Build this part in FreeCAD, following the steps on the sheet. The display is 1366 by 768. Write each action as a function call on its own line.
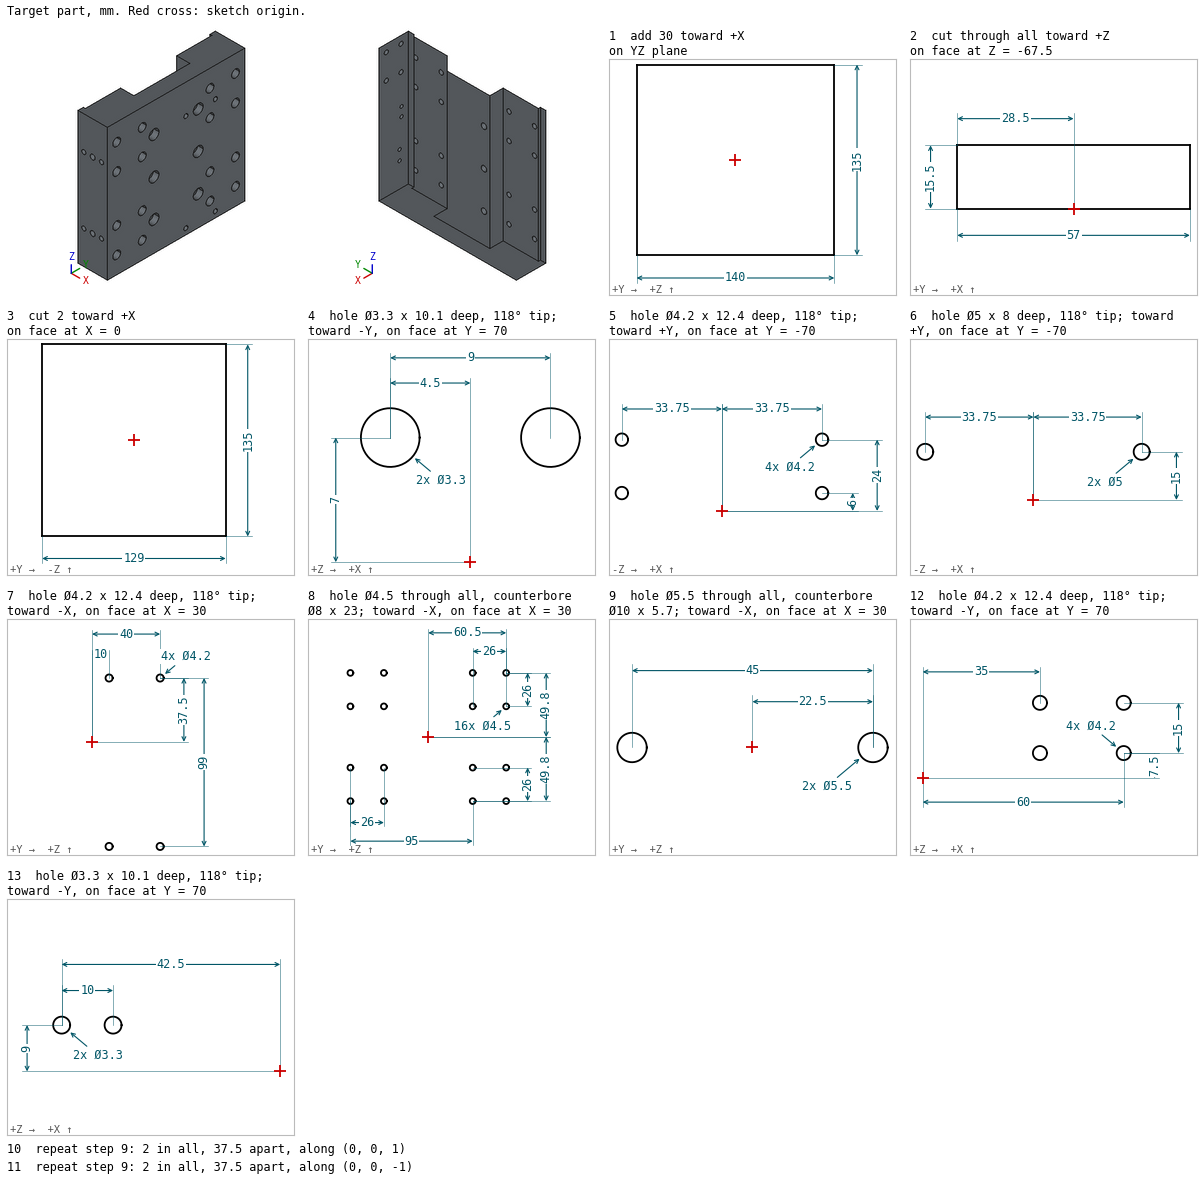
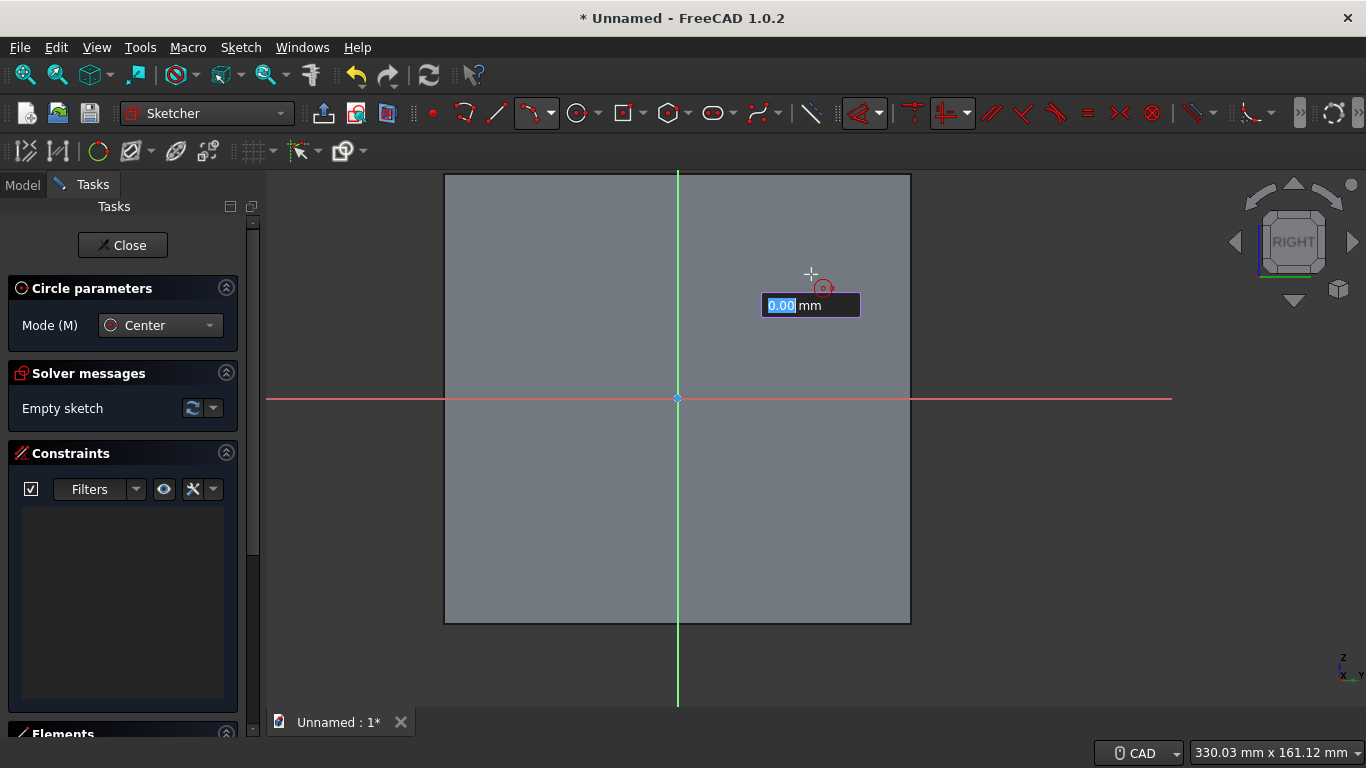
scroll(816, 269, up, 5)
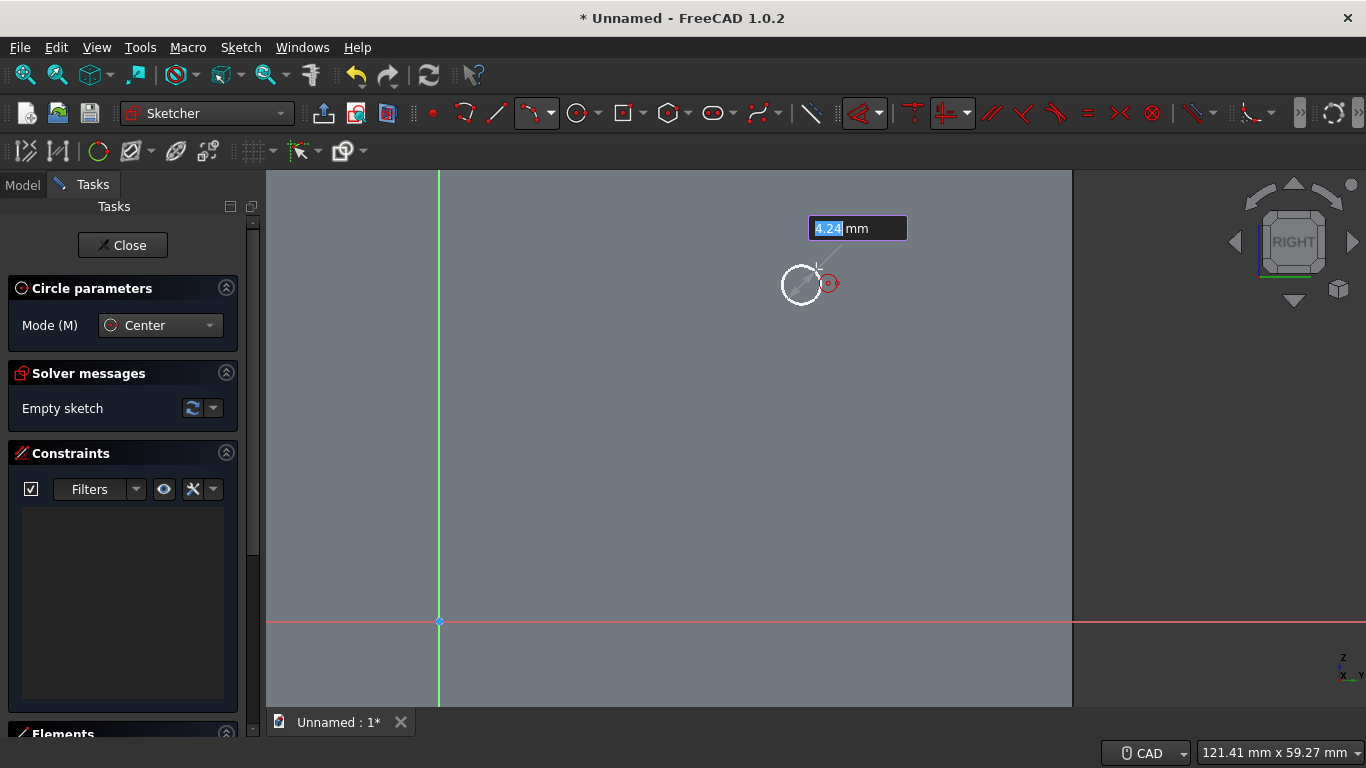
click(815, 268)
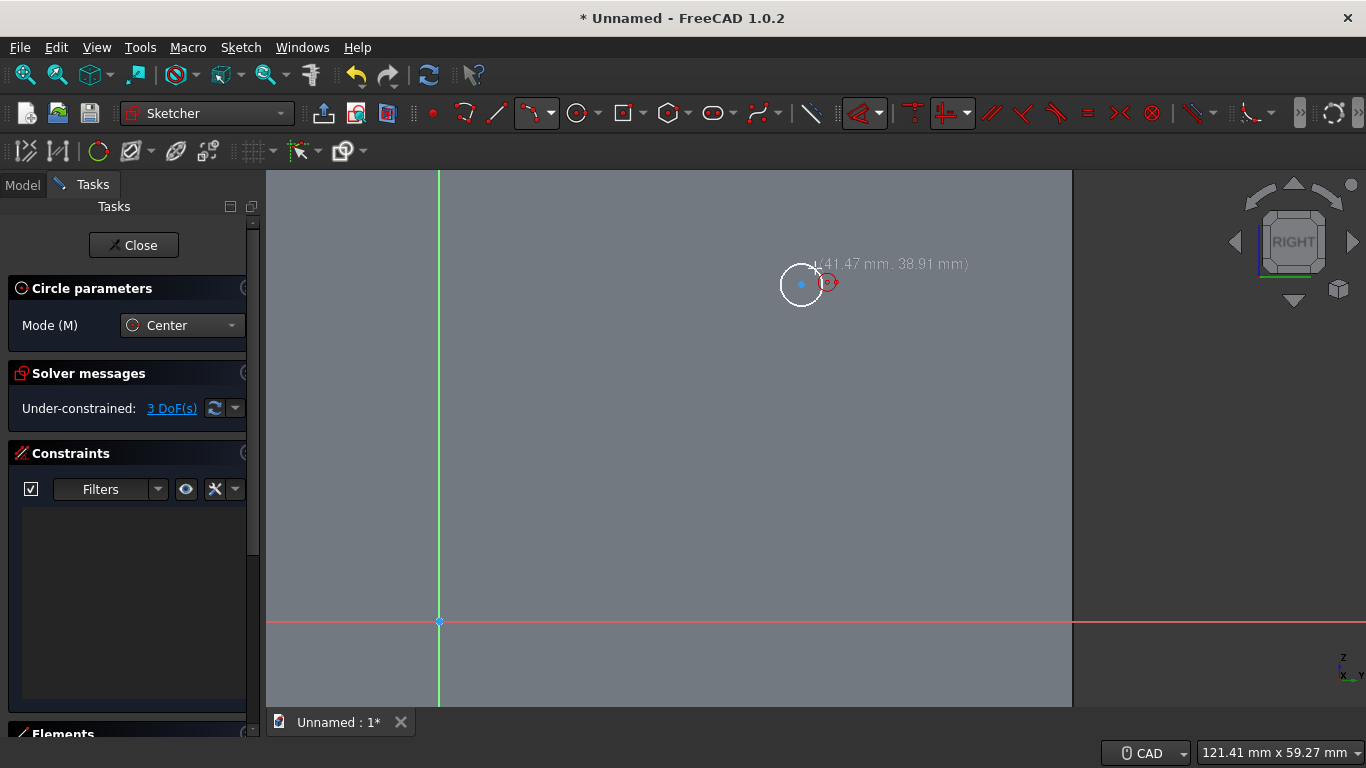
click(530, 282)
click(543, 268)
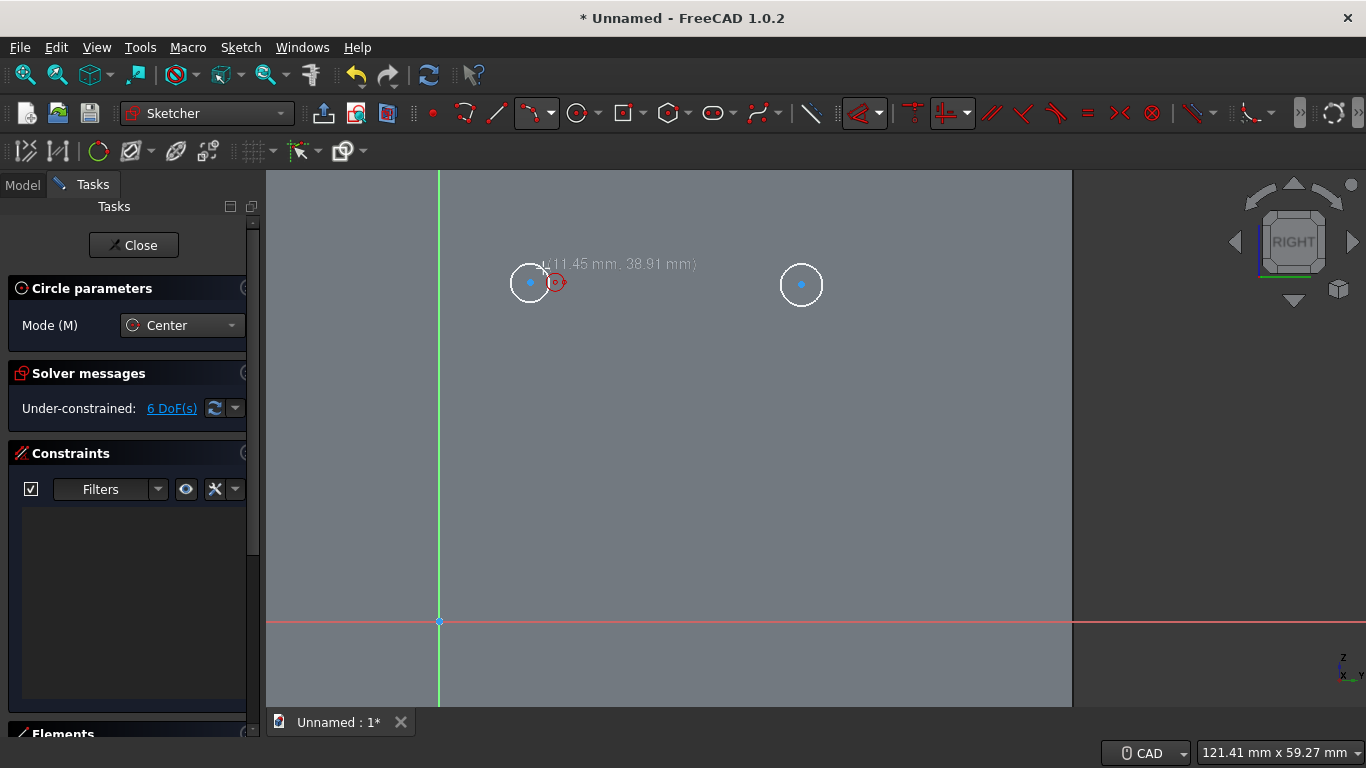
scroll(816, 269, down, 5)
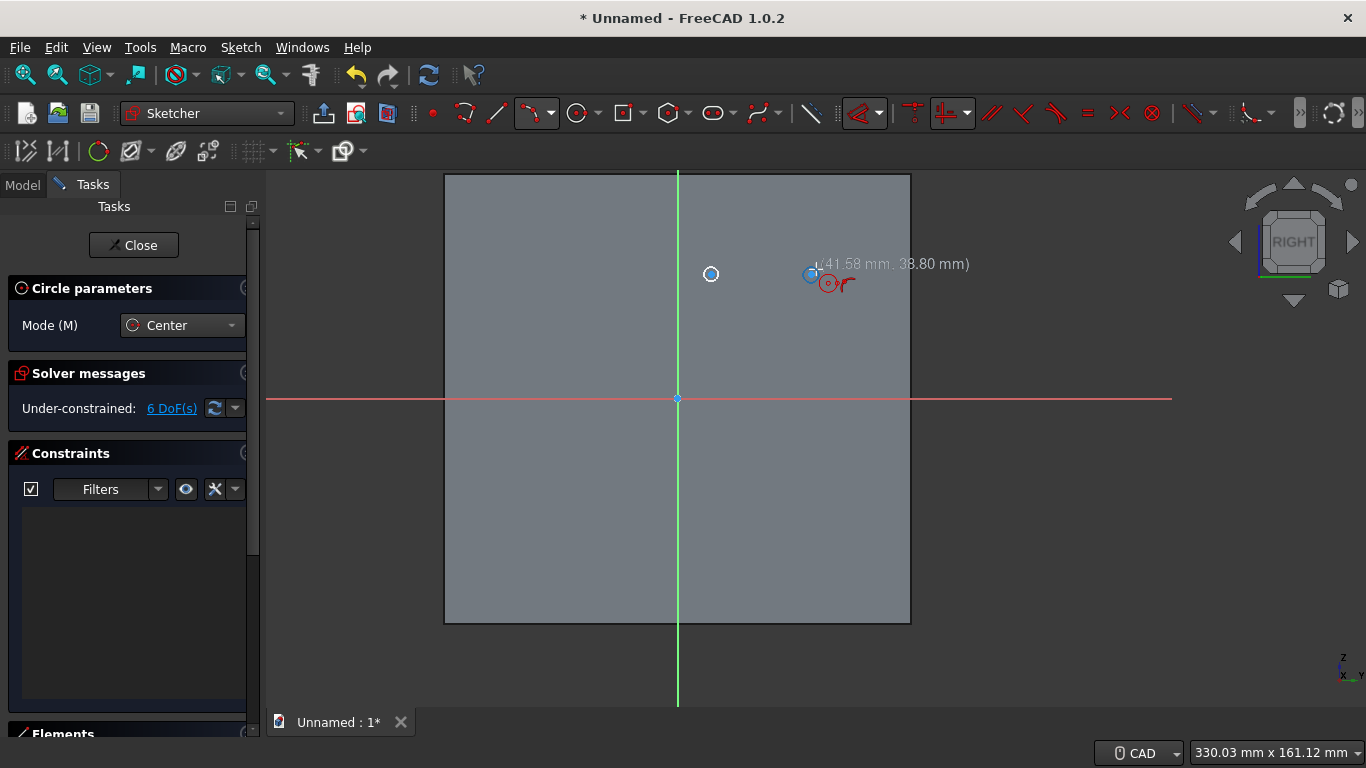
scroll(811, 604, up, 6)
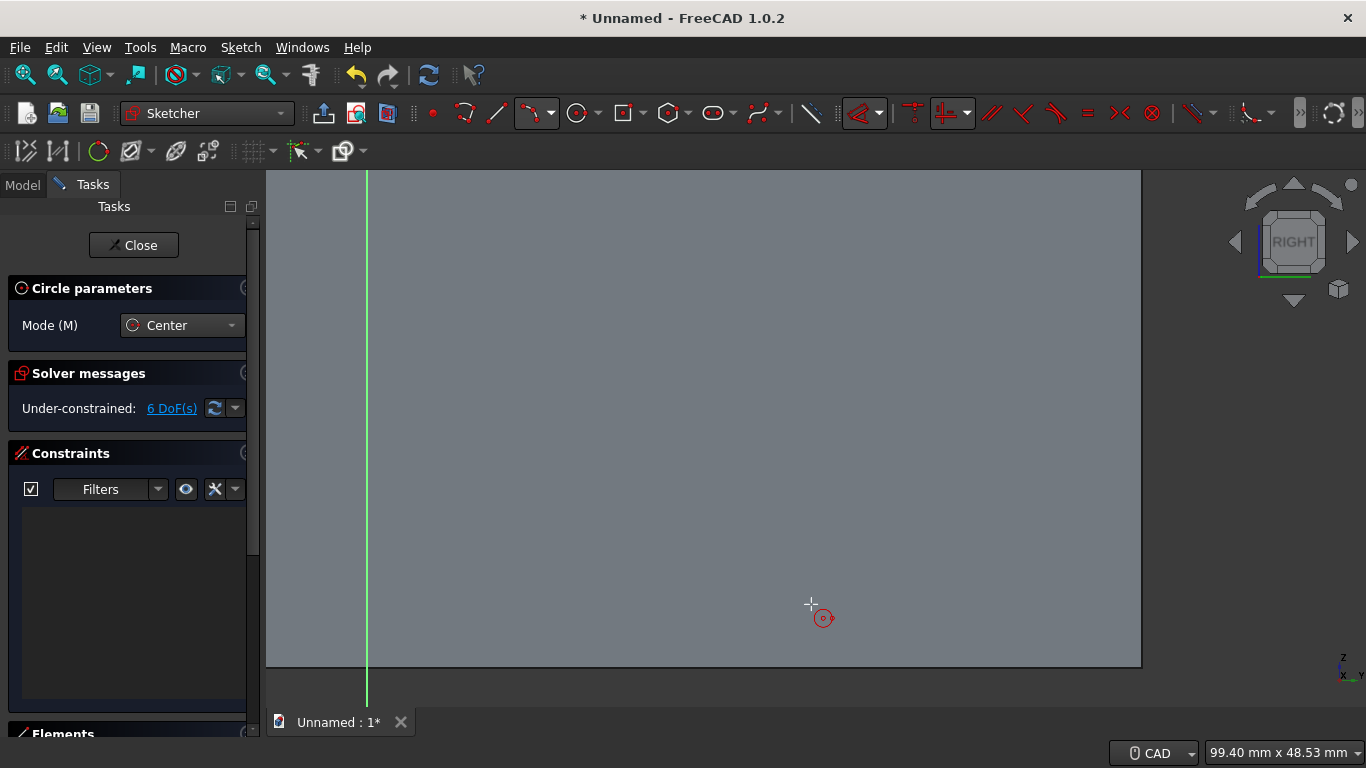
scroll(811, 604, down, 6)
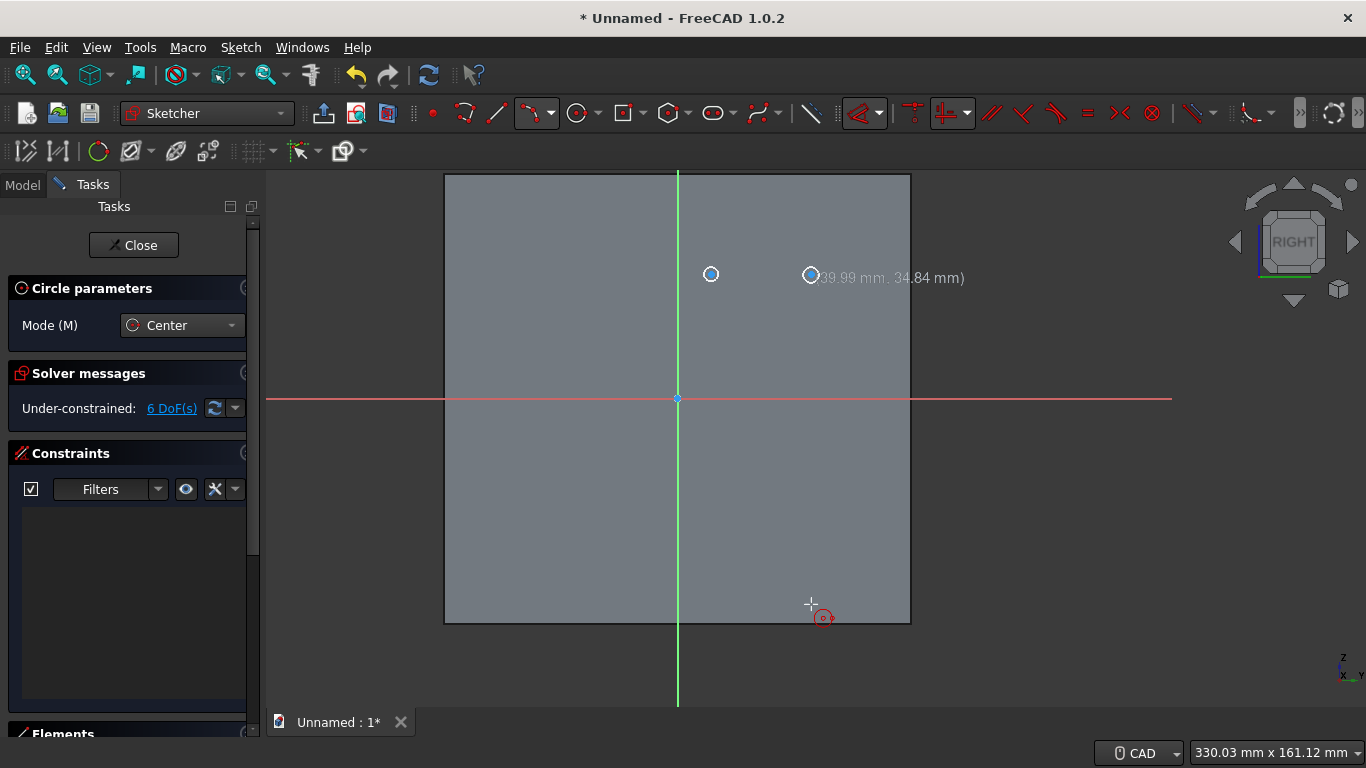
click(811, 604)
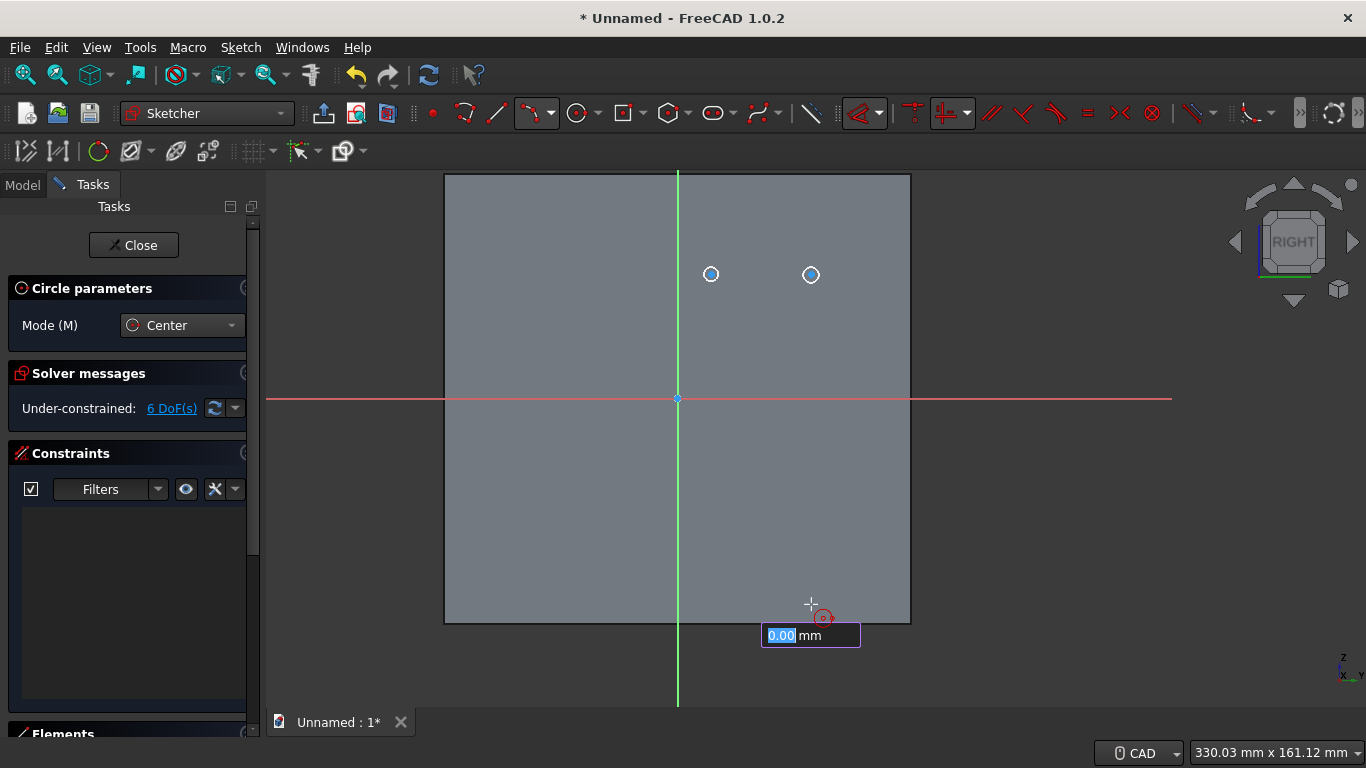
scroll(816, 599, up, 5)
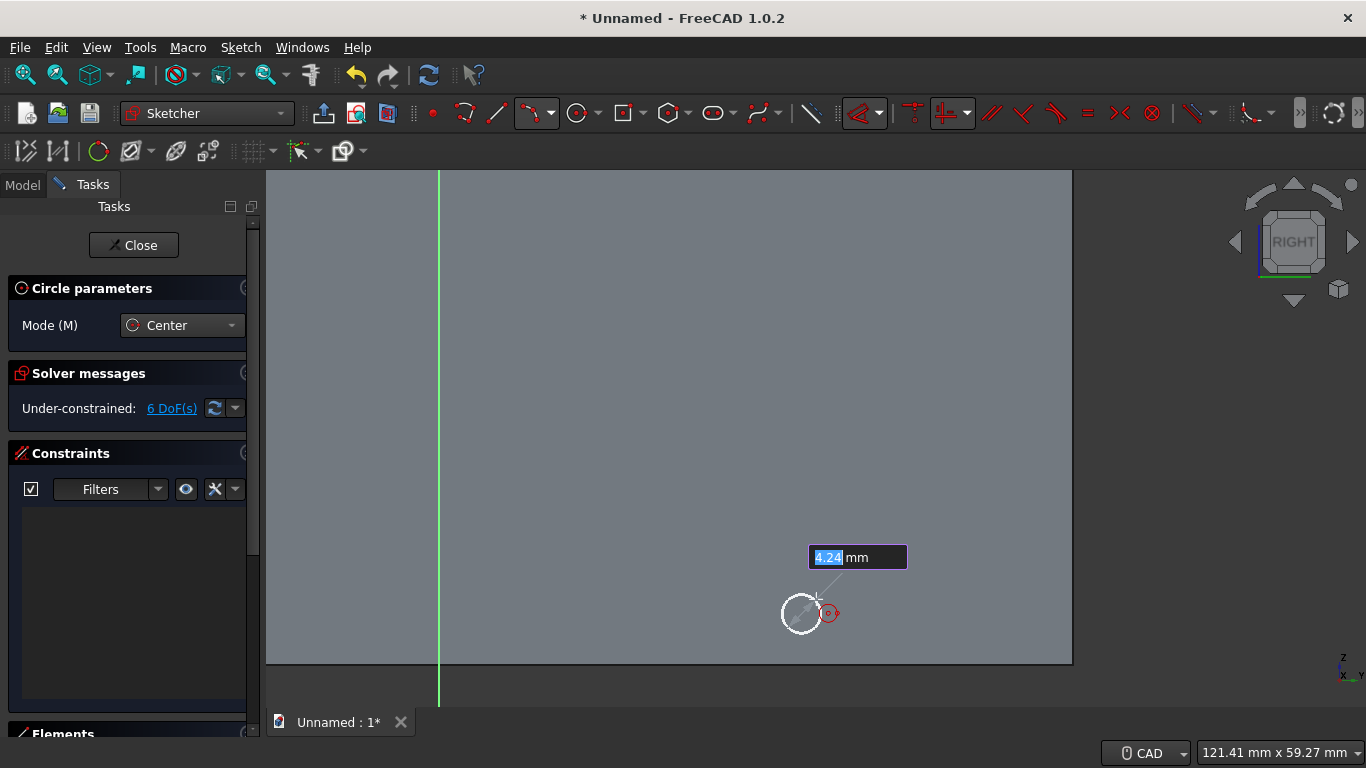
click(815, 597)